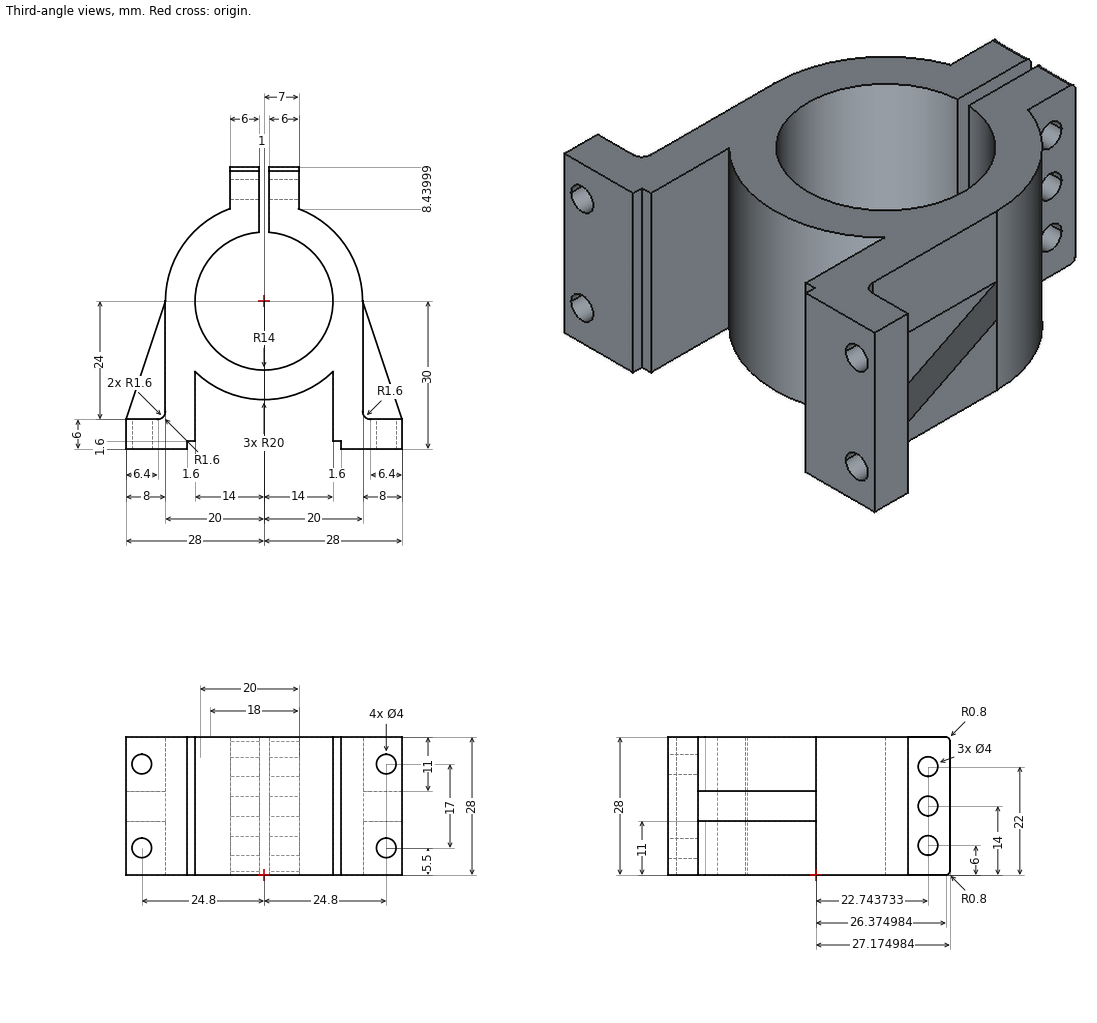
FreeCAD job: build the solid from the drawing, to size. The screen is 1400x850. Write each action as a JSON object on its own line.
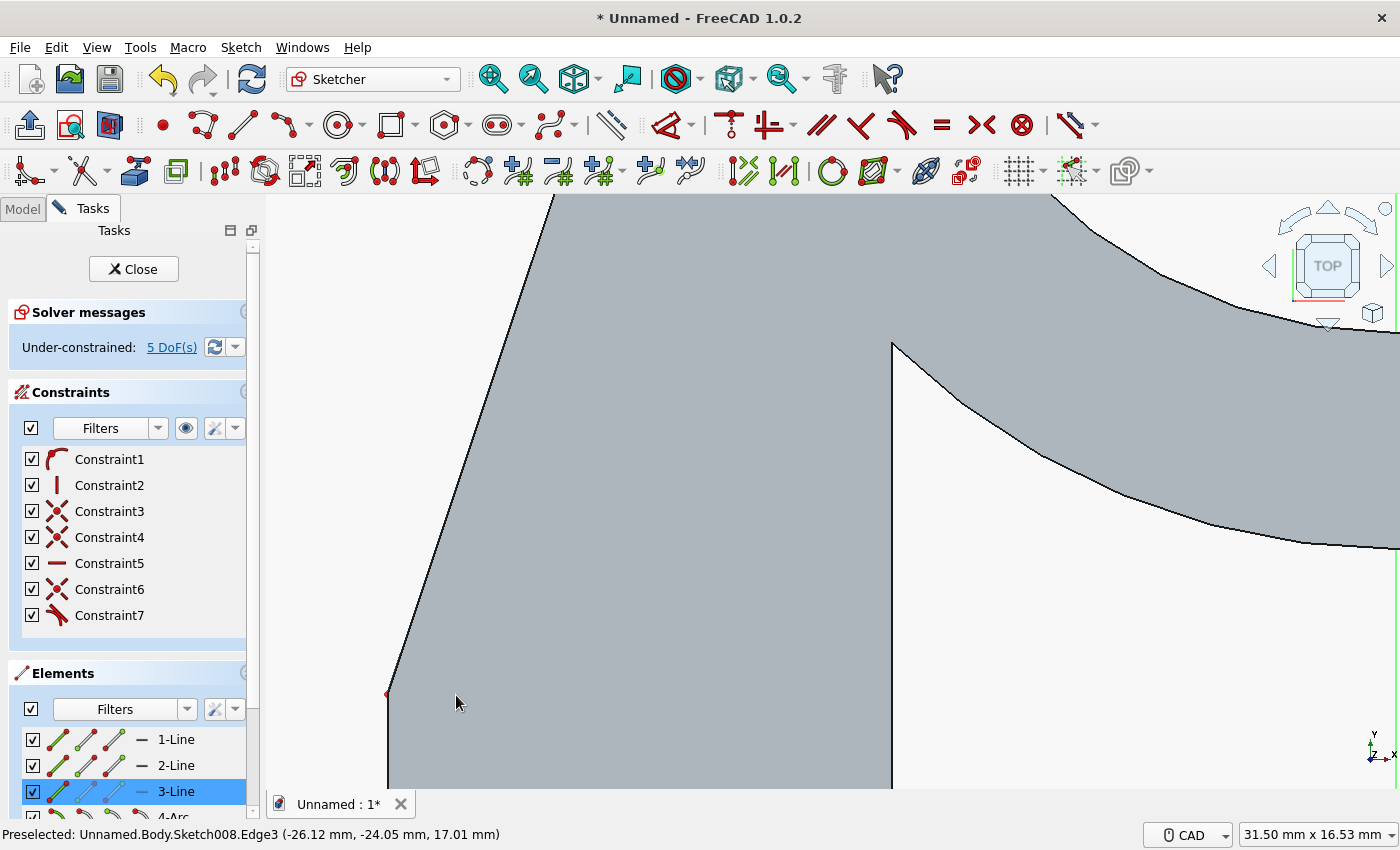
{"action": "left_click", "coordinate": [645, 687]}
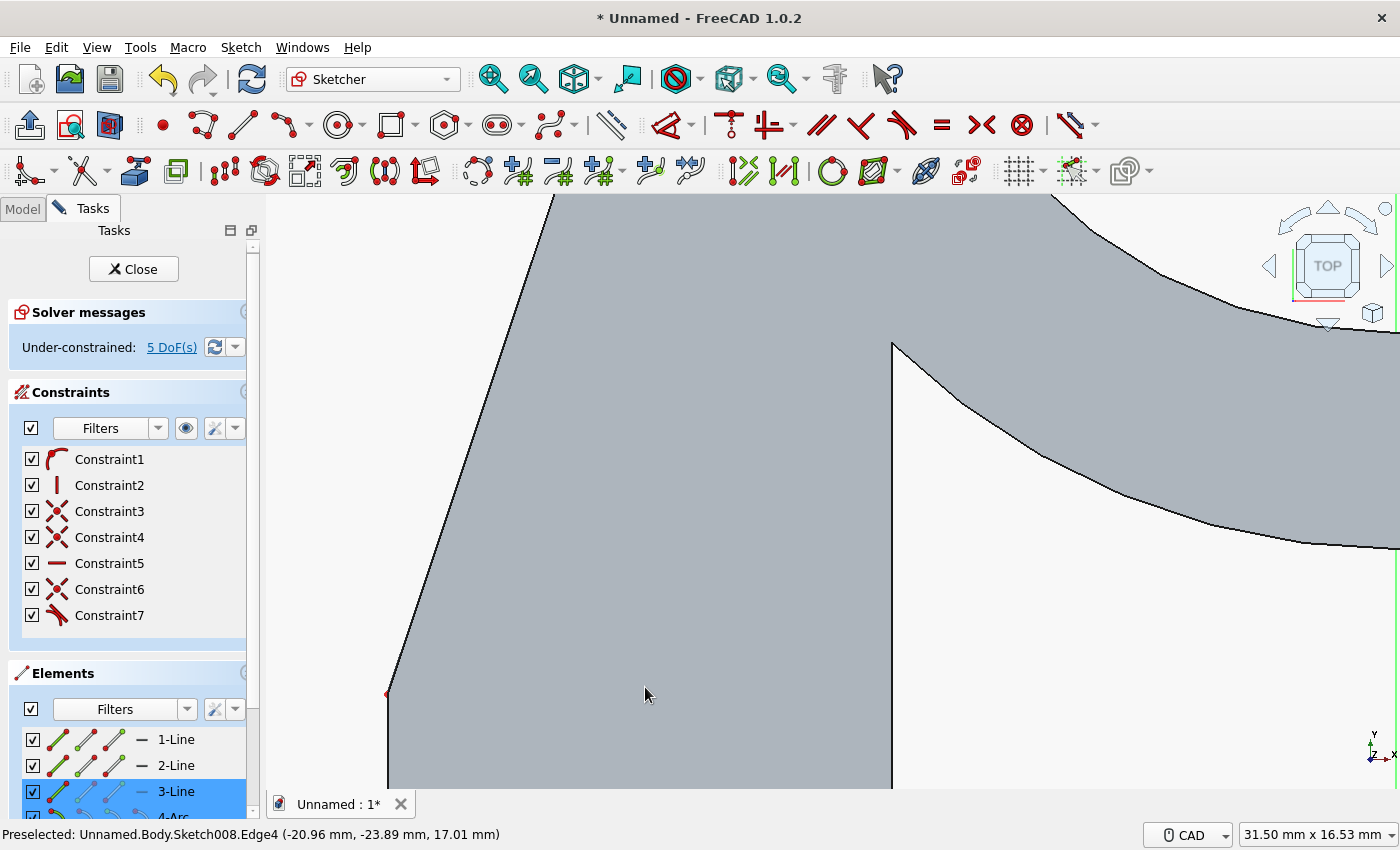
{"action": "left_click", "coordinate": [902, 126]}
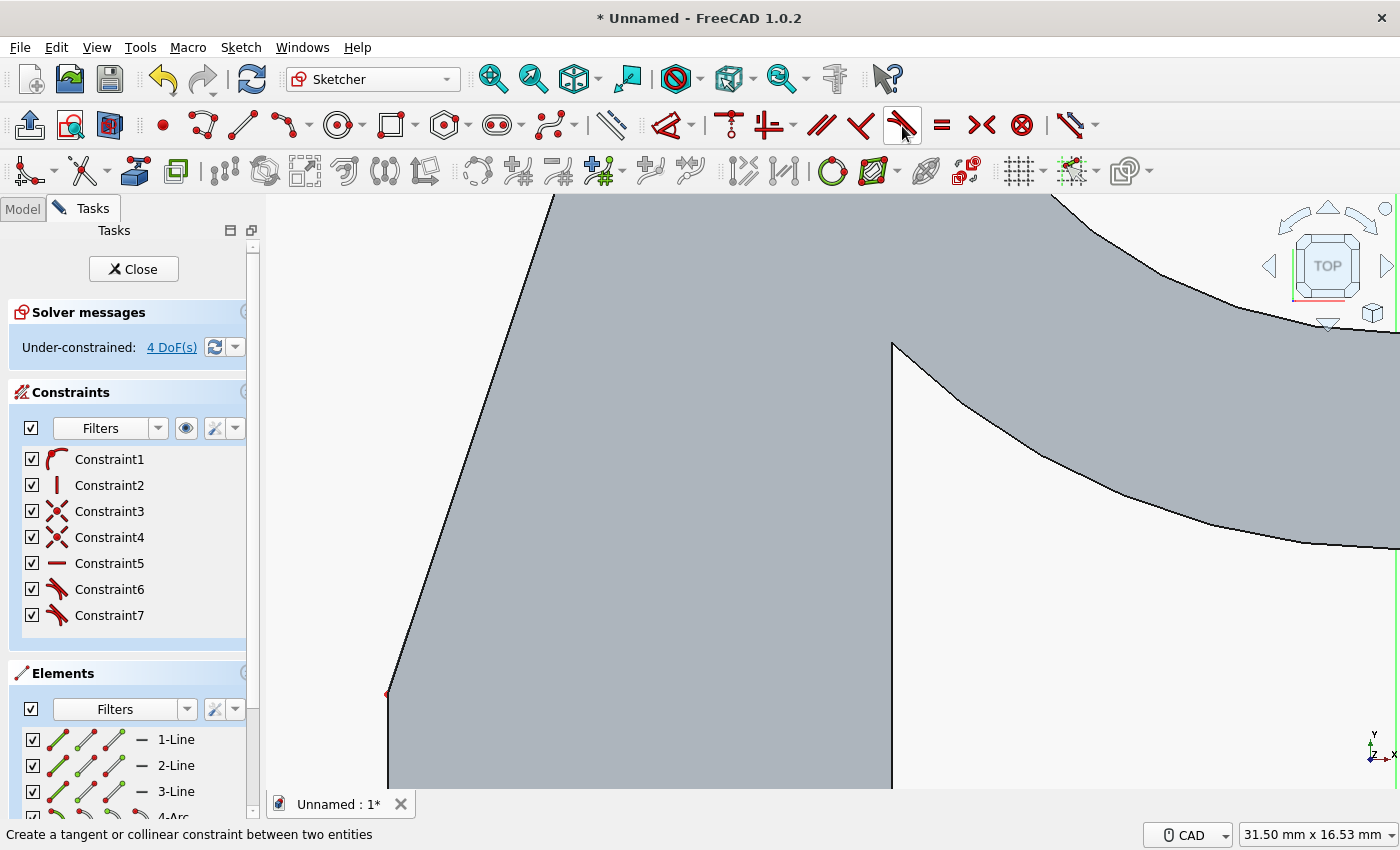
{"action": "left_click", "coordinate": [666, 126]}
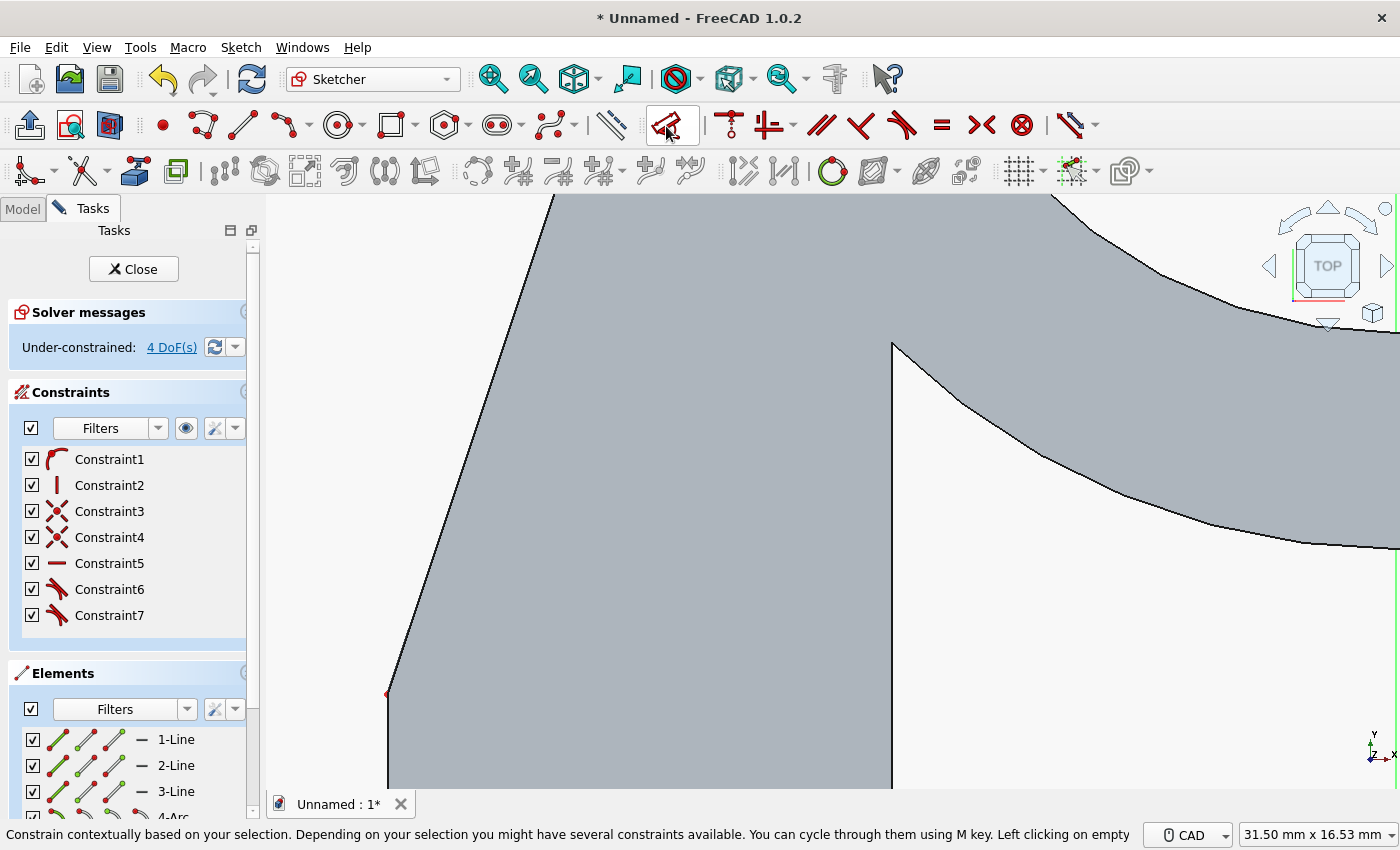
{"action": "left_click", "coordinate": [643, 688]}
{"action": "left_click", "coordinate": [657, 717]}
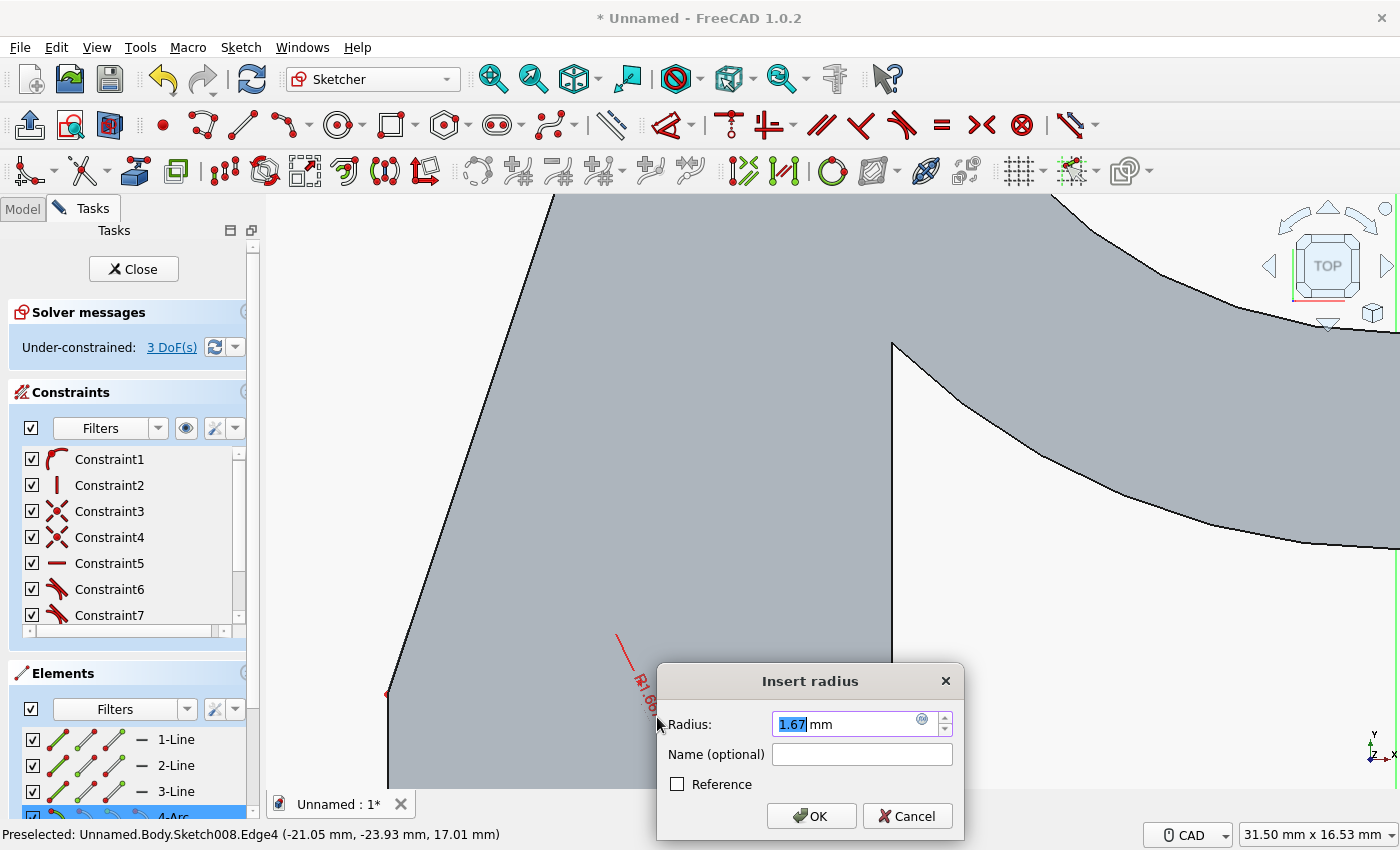
{"action": "type", "text": "1.6"}
{"action": "key", "text": "Return"}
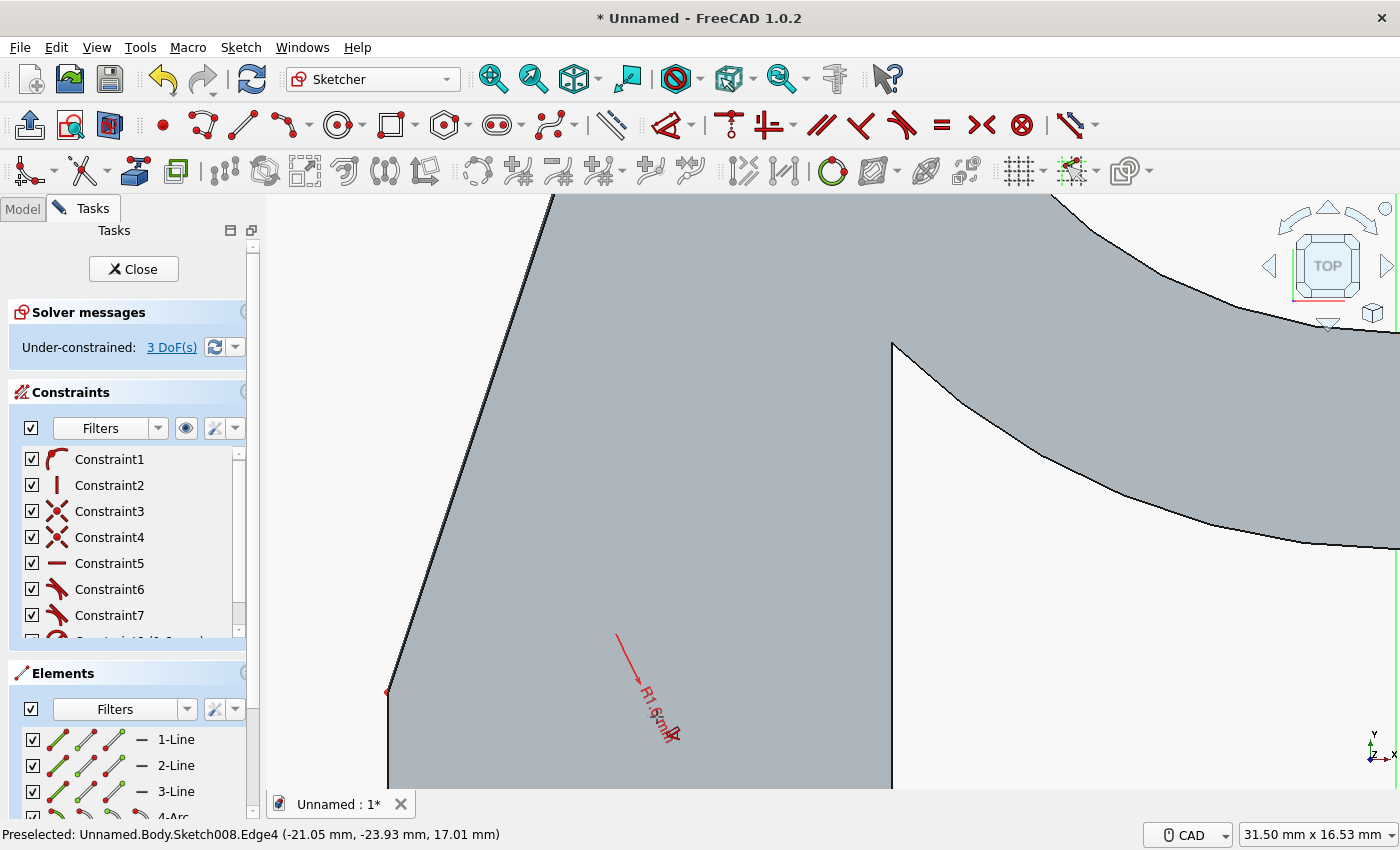
{"action": "left_click", "coordinate": [473, 433]}
{"action": "left_click", "coordinate": [530, 726]}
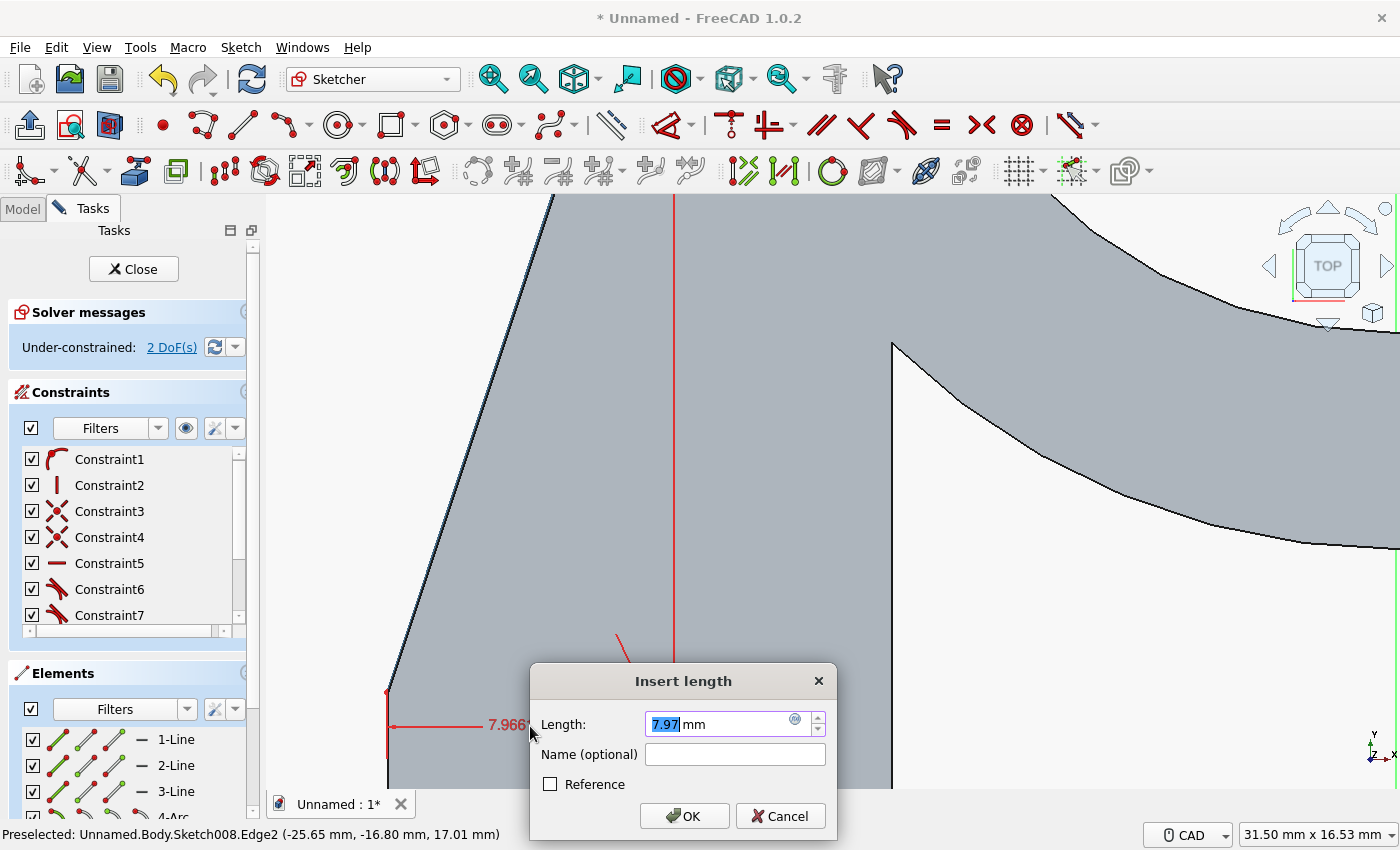
{"action": "type", "text": "8"}
{"action": "key", "text": "Return"}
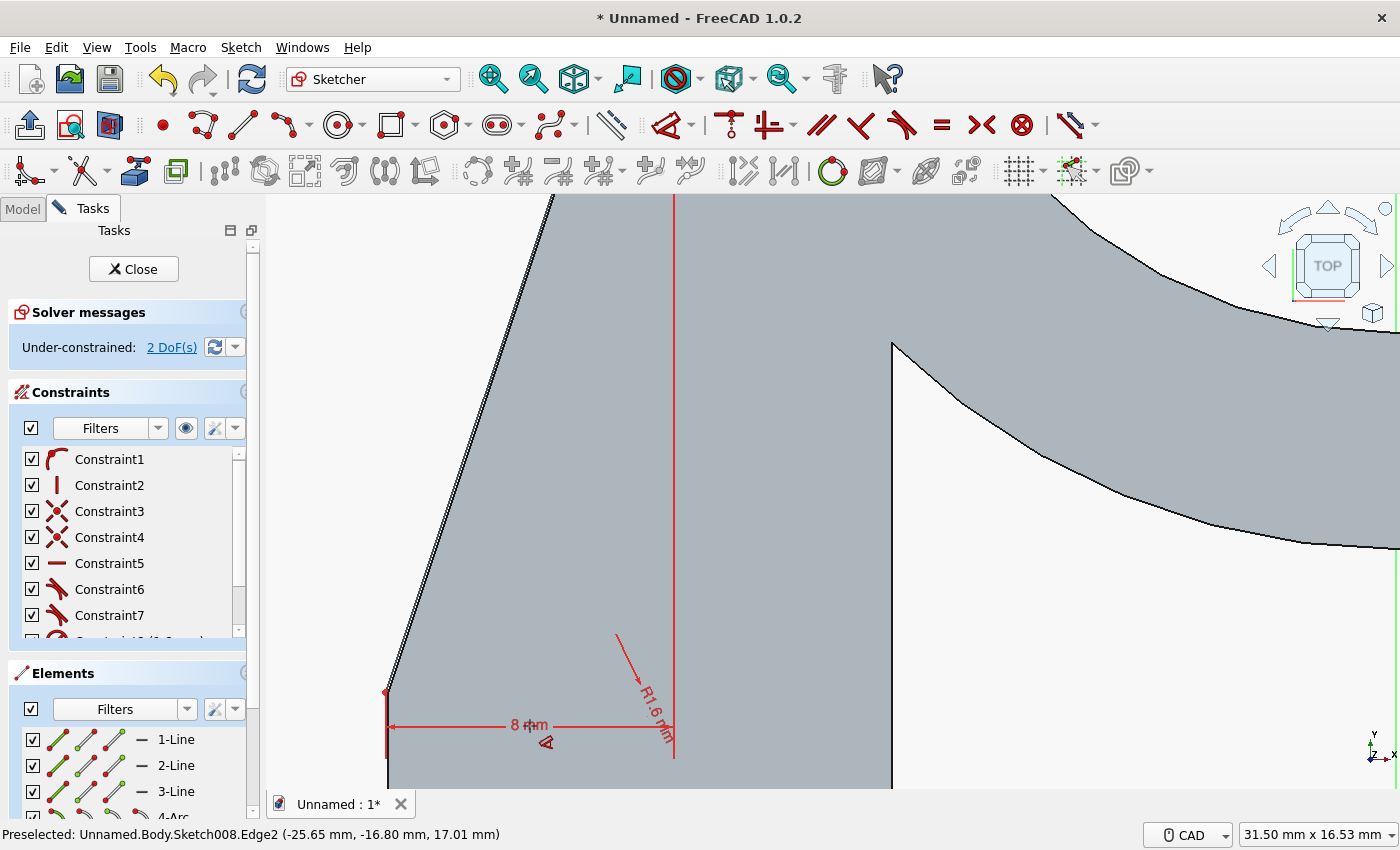
{"action": "left_click", "coordinate": [674, 635]}
{"action": "left_click", "coordinate": [954, 669]}